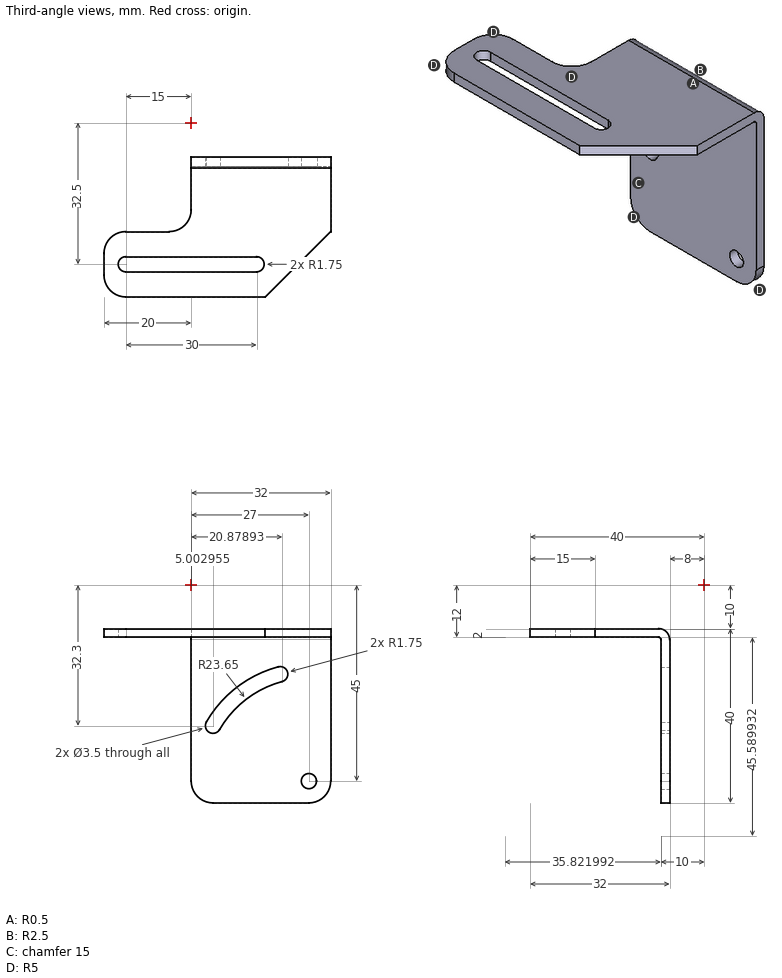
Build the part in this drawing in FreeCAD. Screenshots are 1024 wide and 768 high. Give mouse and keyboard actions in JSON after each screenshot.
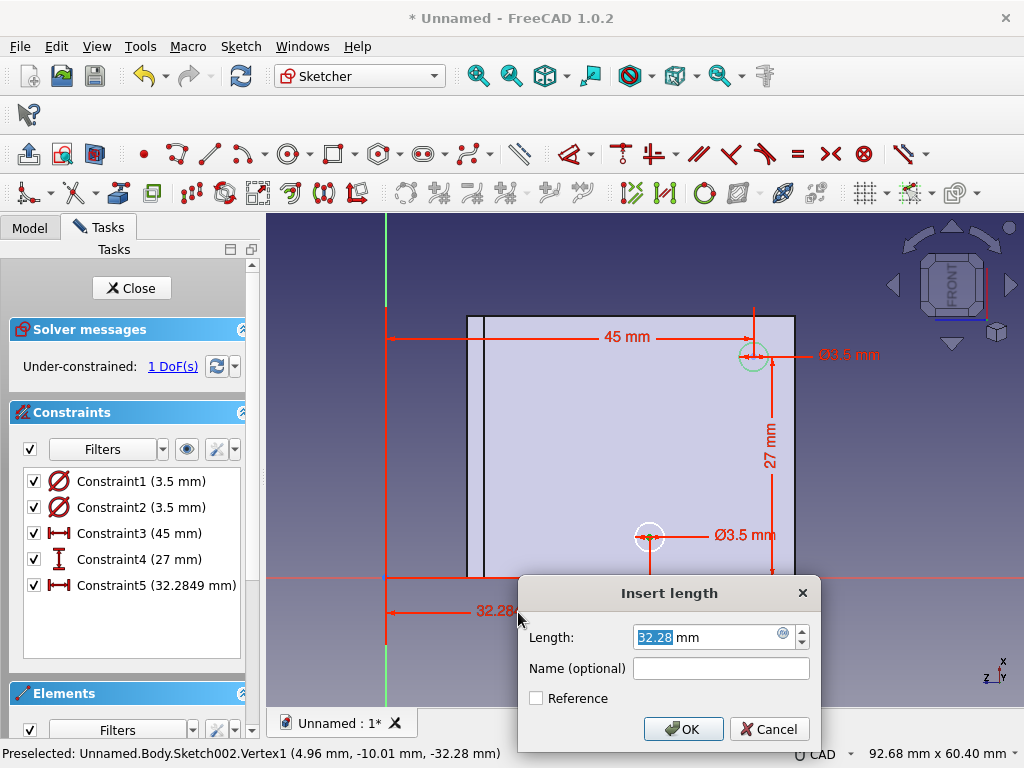
{"action": "type", "text": "32.3"}
{"action": "key", "text": "Return"}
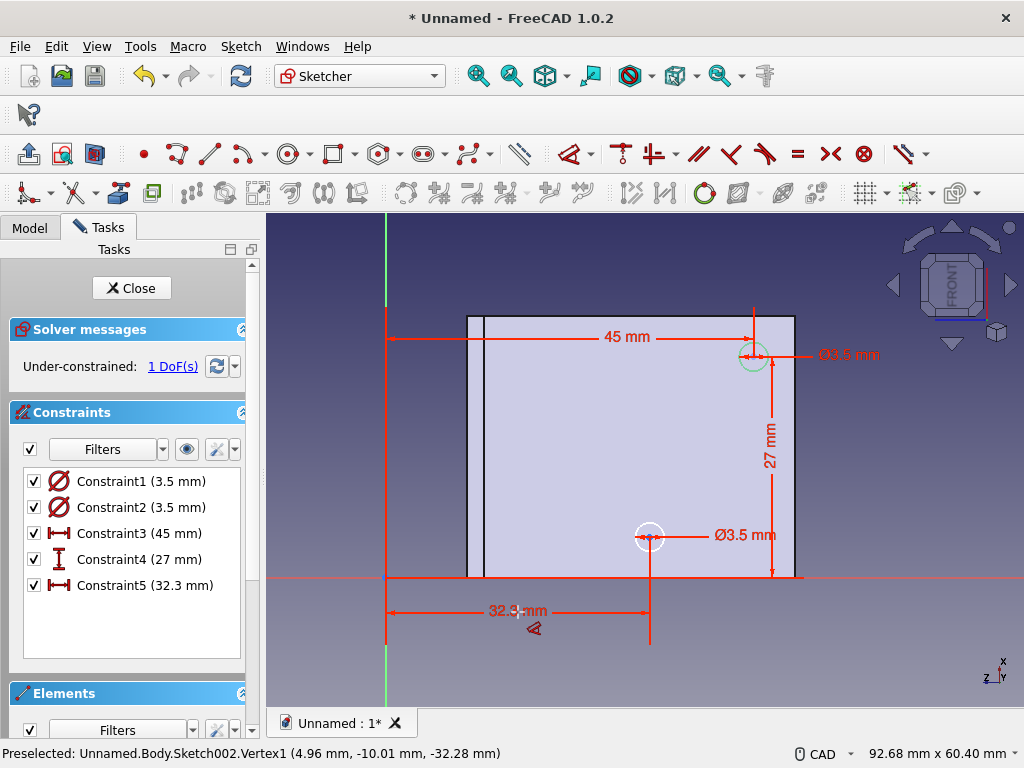
{"action": "left_click", "coordinate": [650, 537]}
{"action": "left_click", "coordinate": [352, 557]}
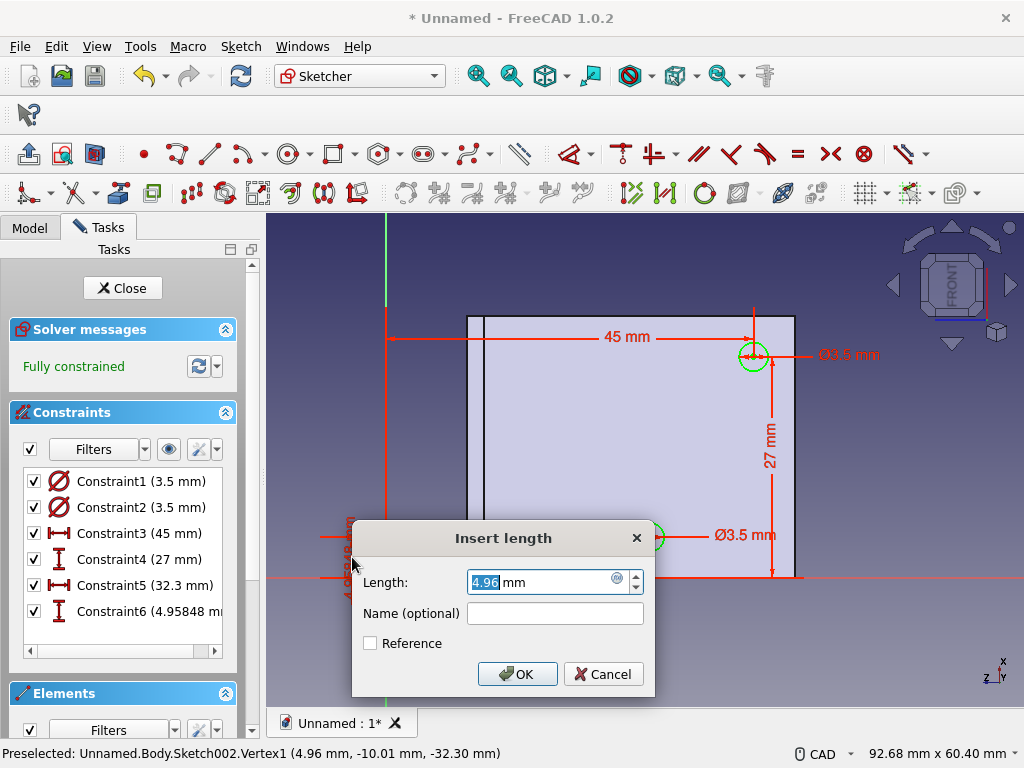
{"action": "type", "text": "5.002955"}
{"action": "key", "text": "Return"}
{"action": "key", "text": "Escape"}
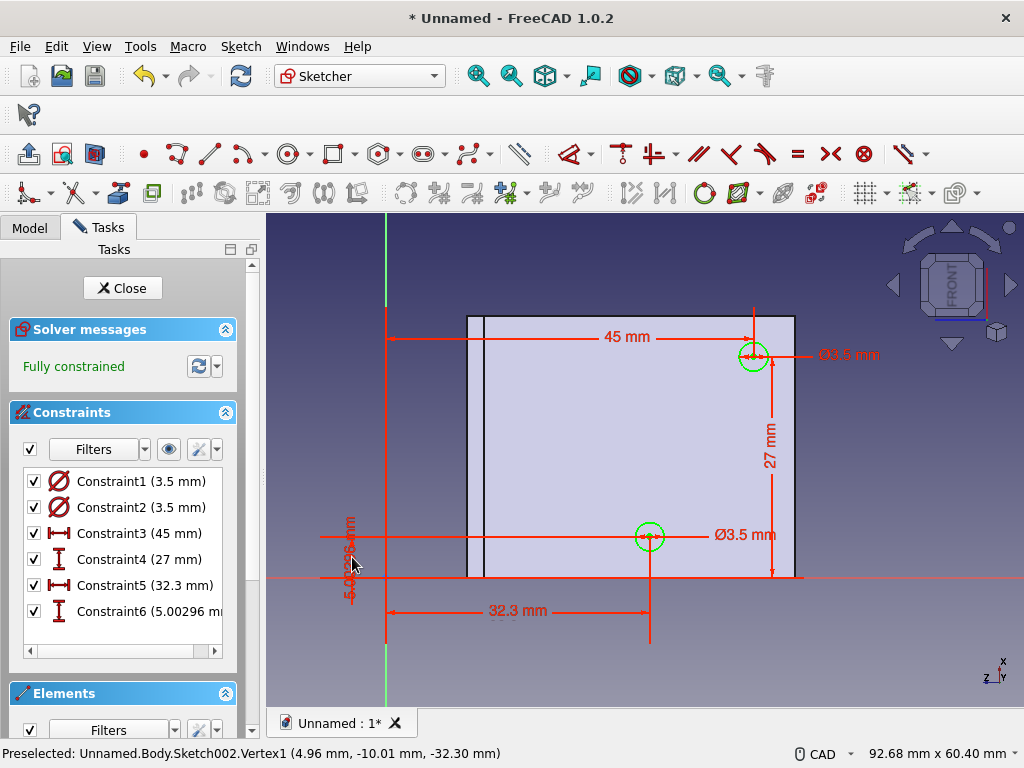
{"action": "left_click", "coordinate": [123, 288]}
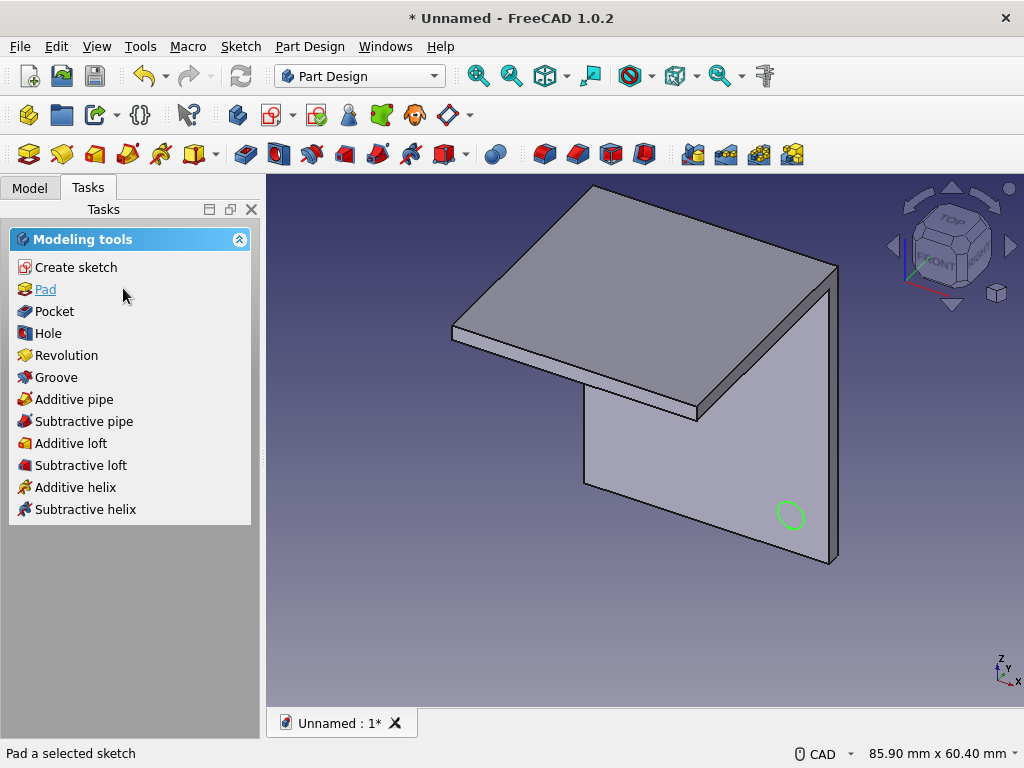
{"action": "left_click", "coordinate": [279, 154]}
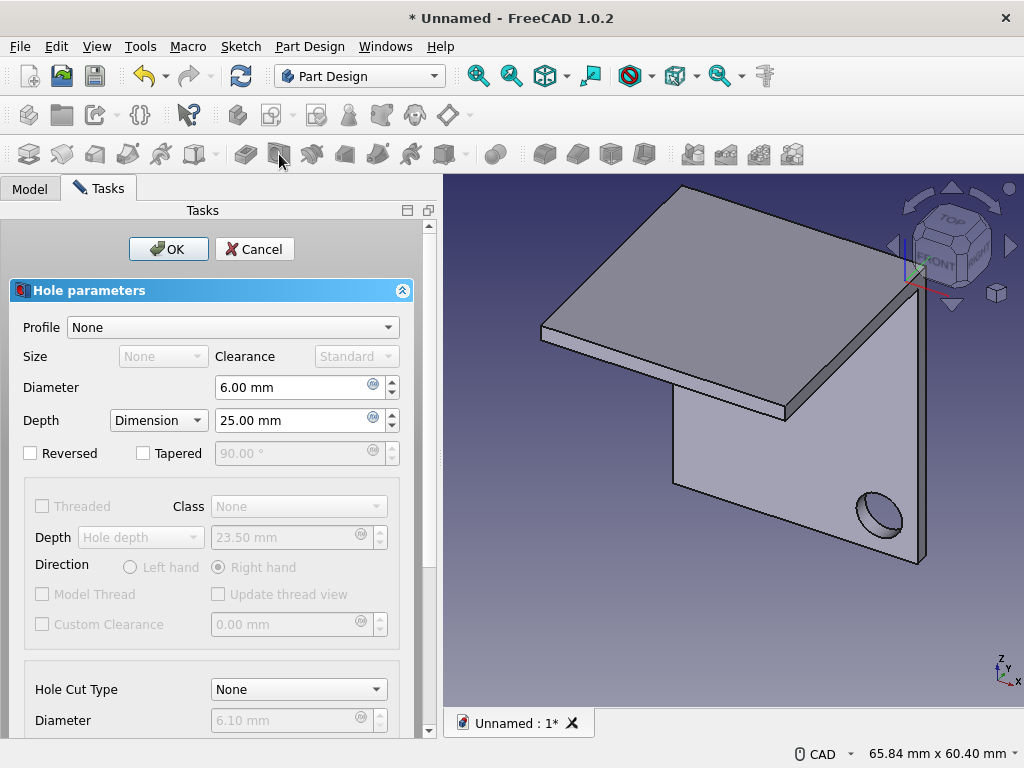
{"action": "triple_click", "coordinate": [300, 388]}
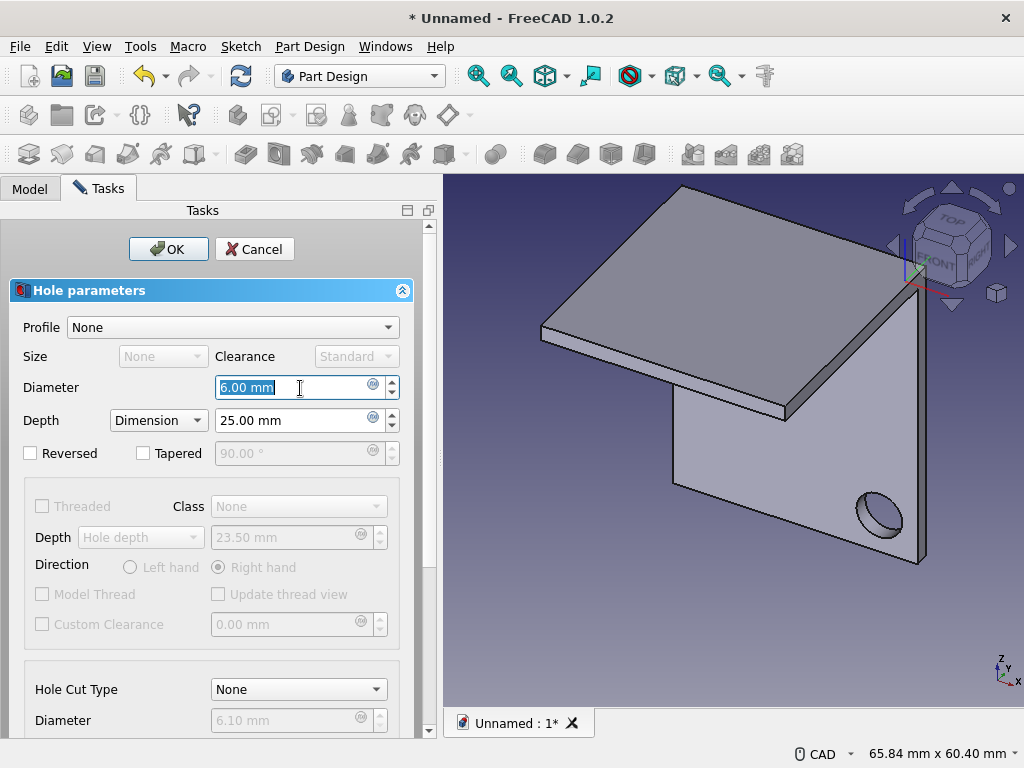
{"action": "type", "text": "3.5"}
{"action": "key", "text": "Tab"}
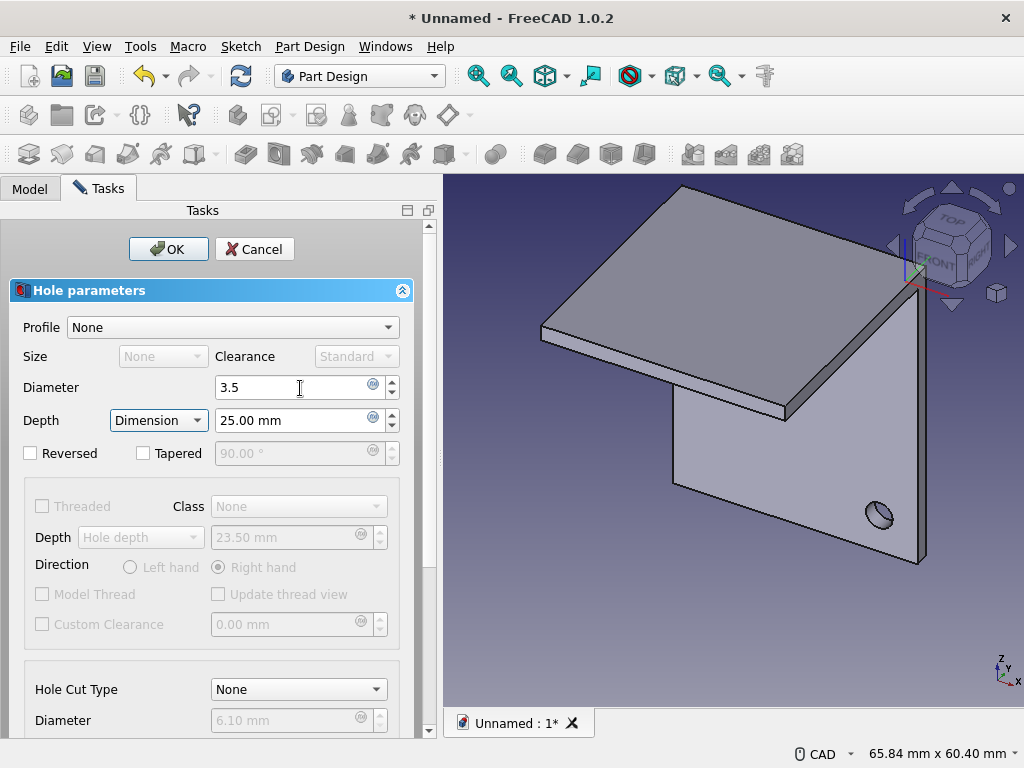
{"action": "left_click", "coordinate": [160, 420]}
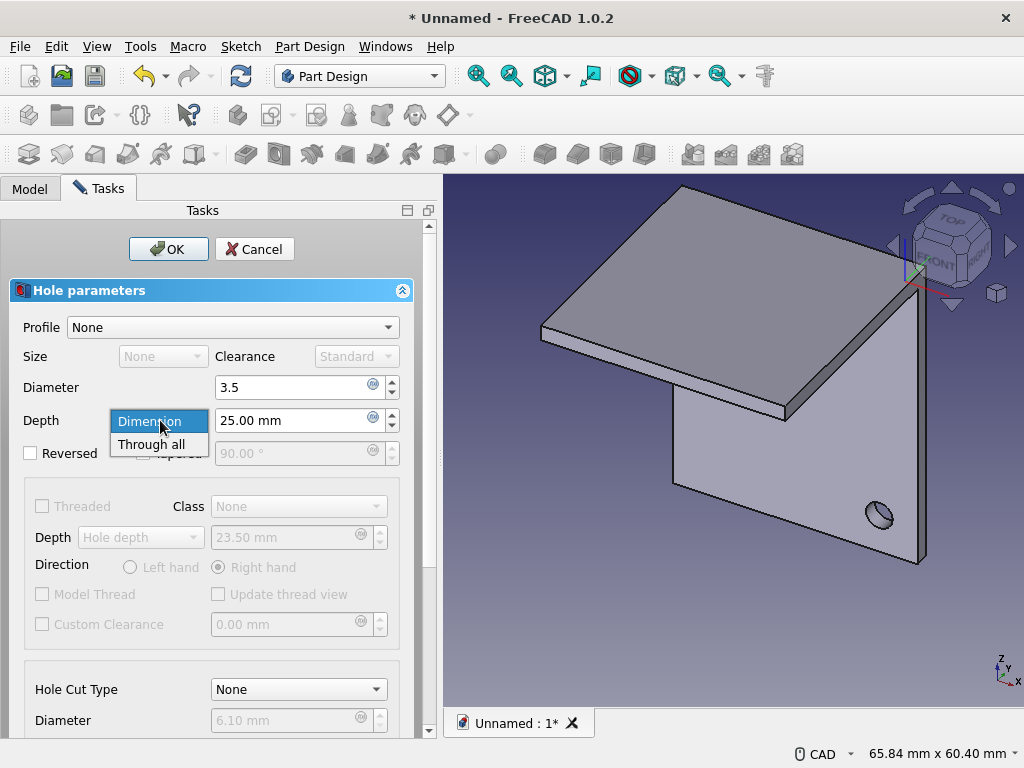
{"action": "left_click", "coordinate": [158, 444]}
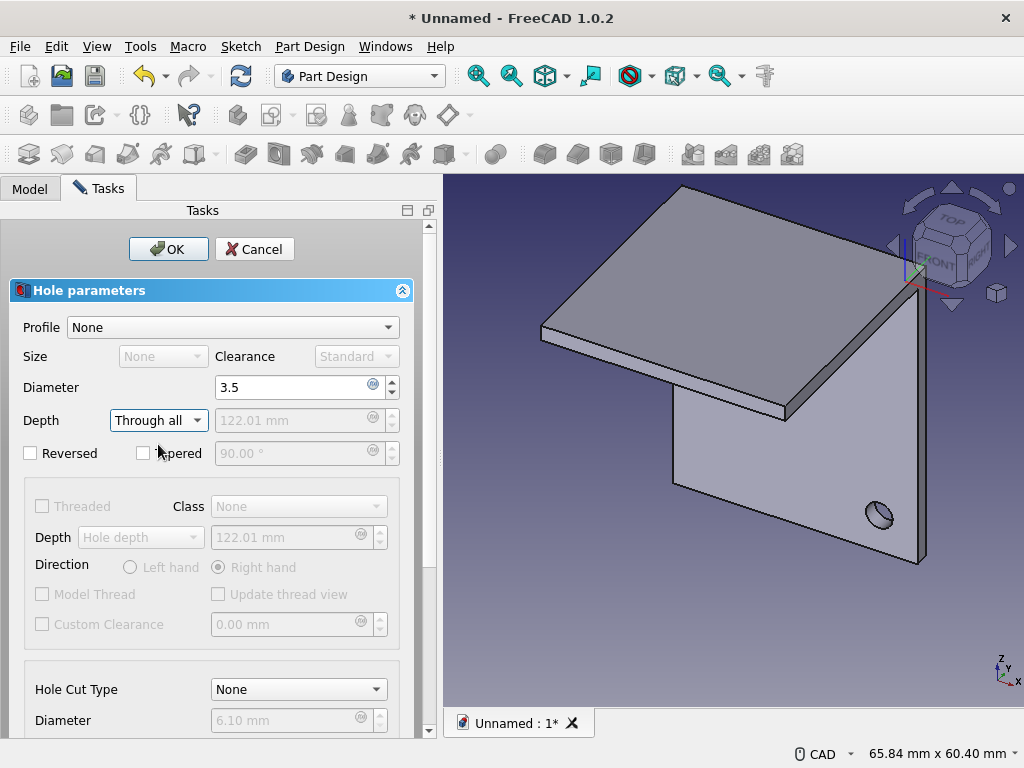
{"action": "left_click", "coordinate": [169, 249]}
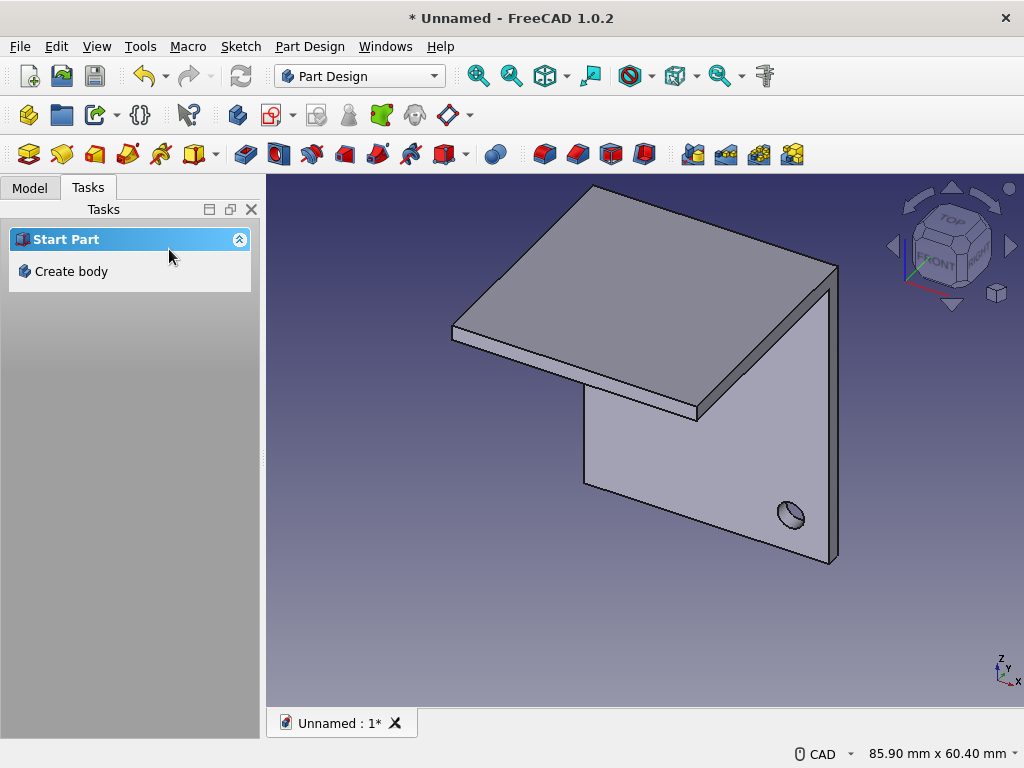
{"action": "key", "text": "0"}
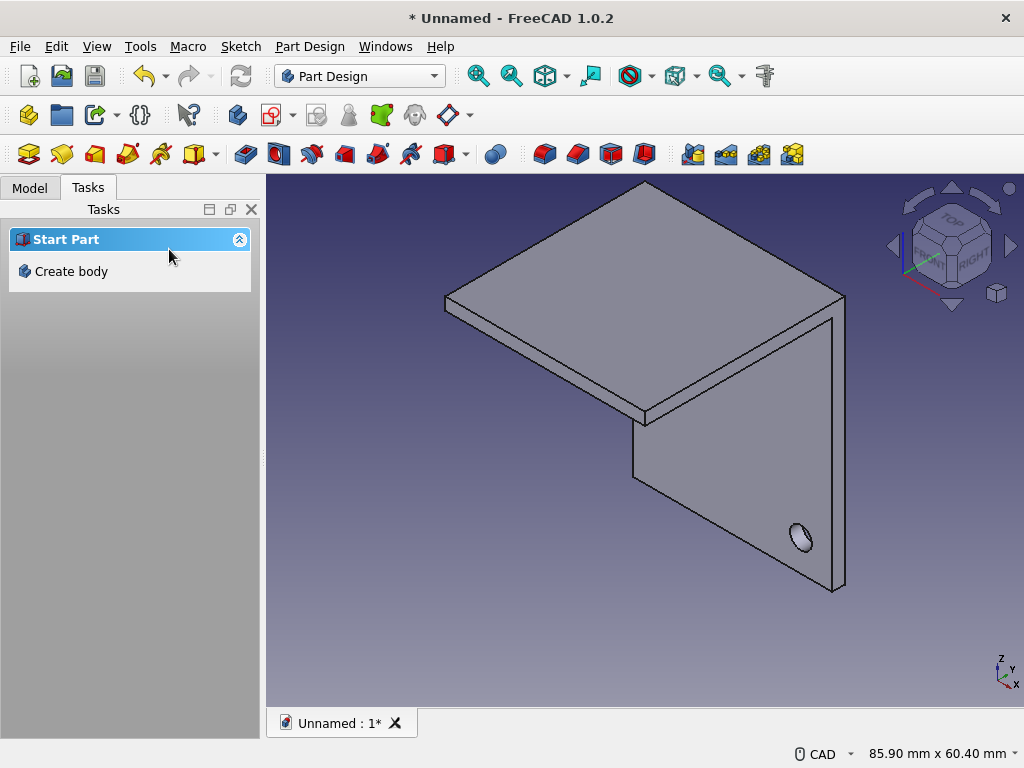
{"action": "key", "text": "2"}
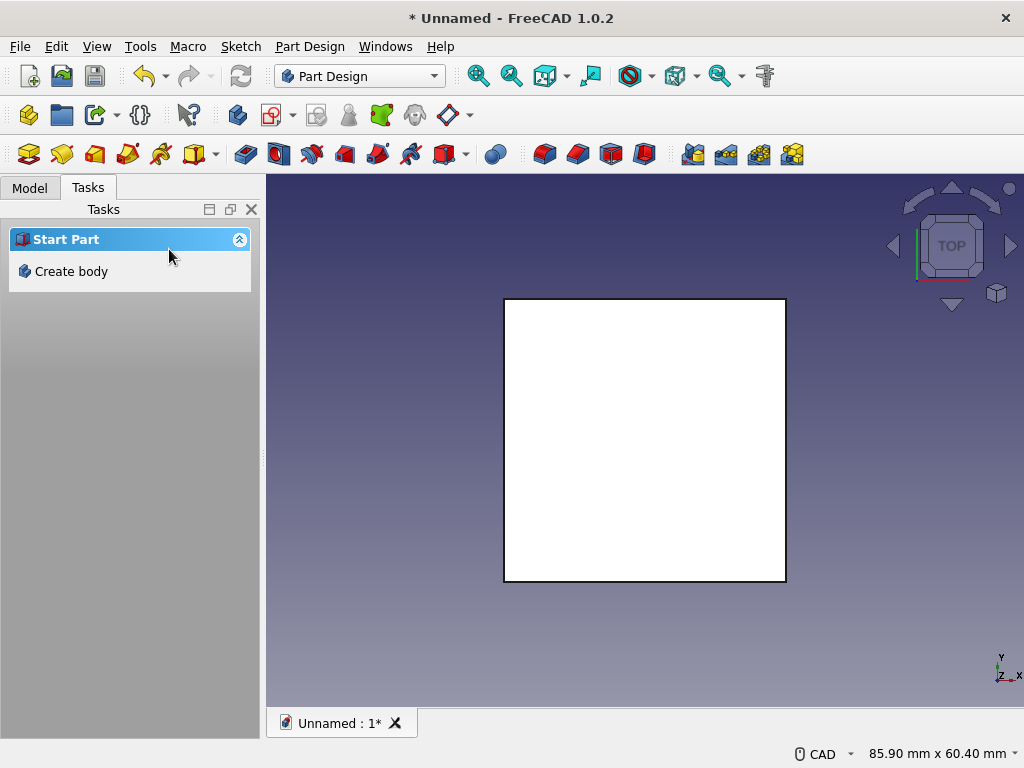
{"action": "key", "text": "1"}